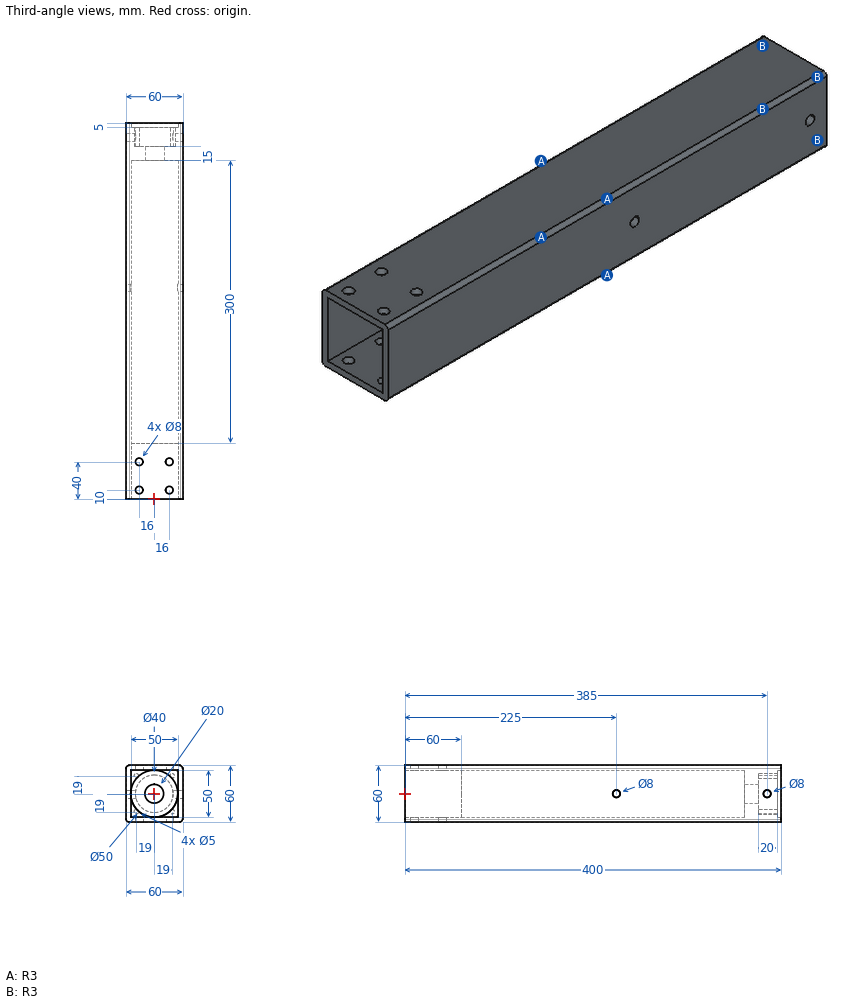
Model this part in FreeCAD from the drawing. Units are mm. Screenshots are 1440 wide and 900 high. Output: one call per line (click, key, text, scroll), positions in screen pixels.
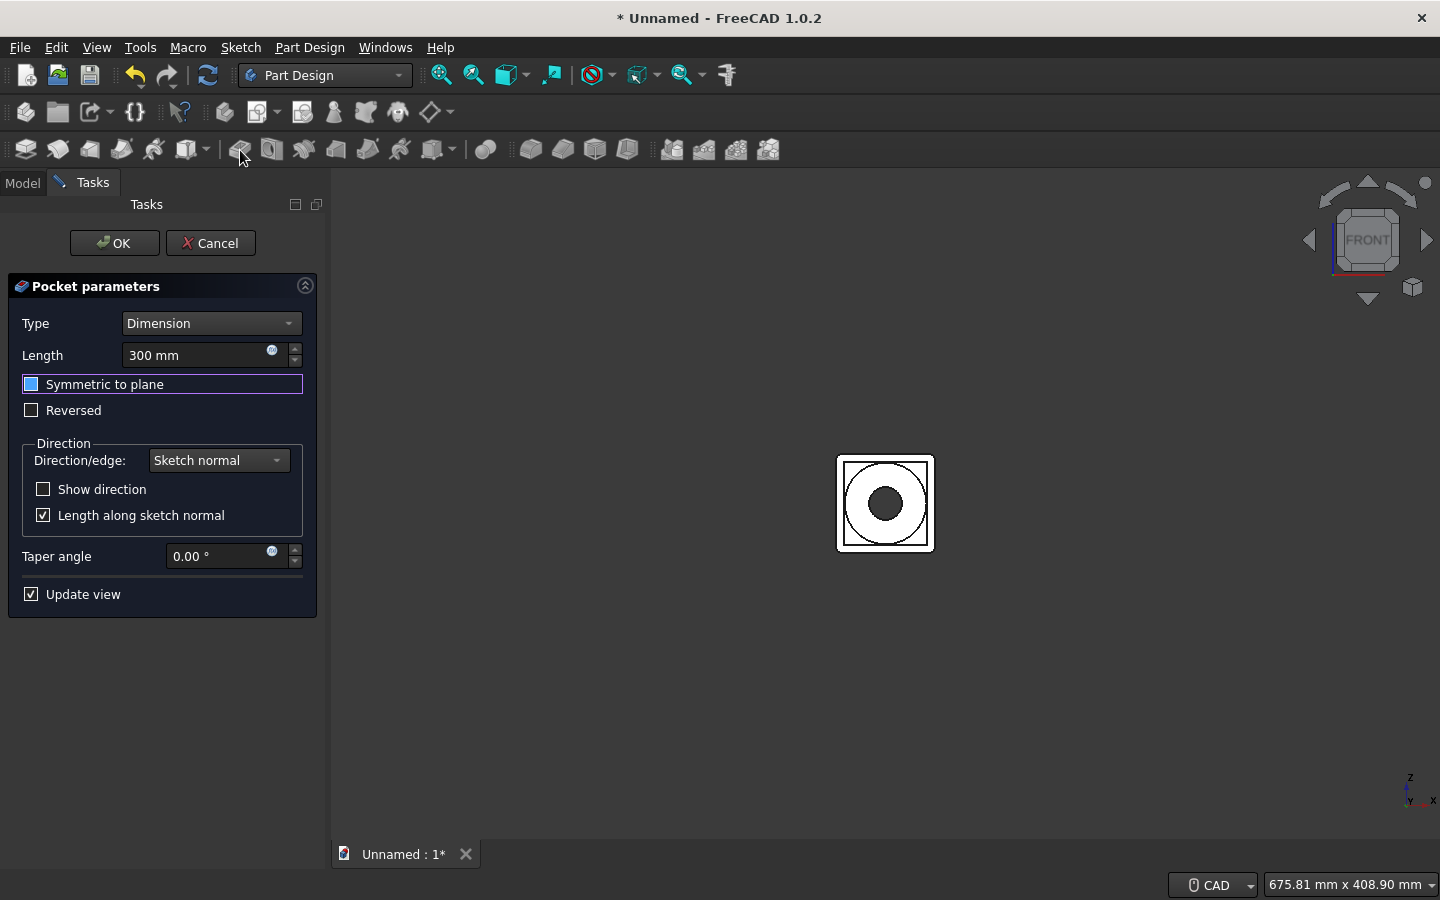
click(115, 243)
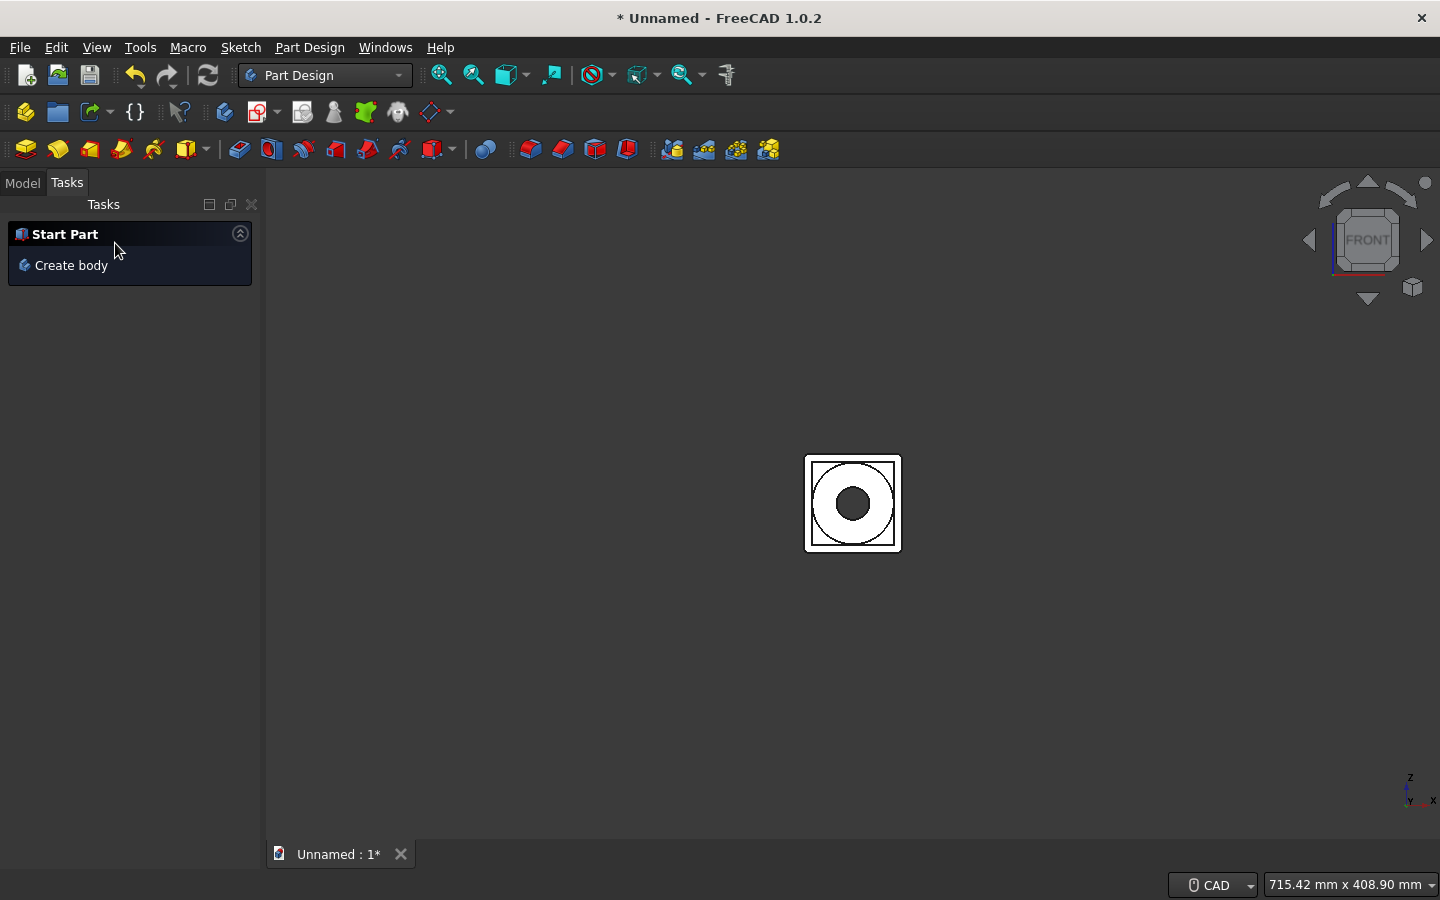
click(442, 76)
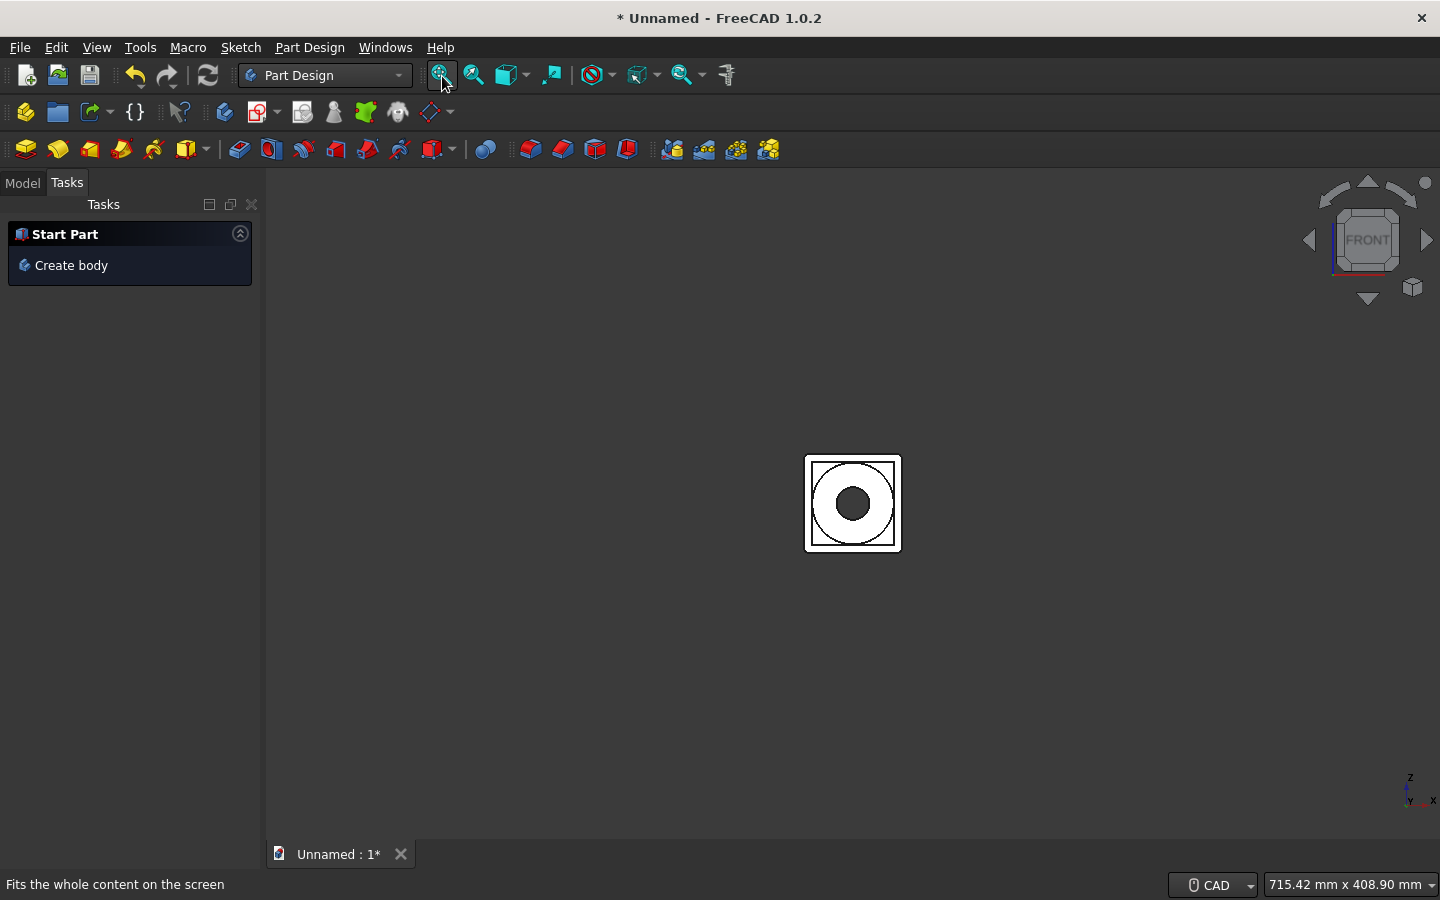
click(258, 112)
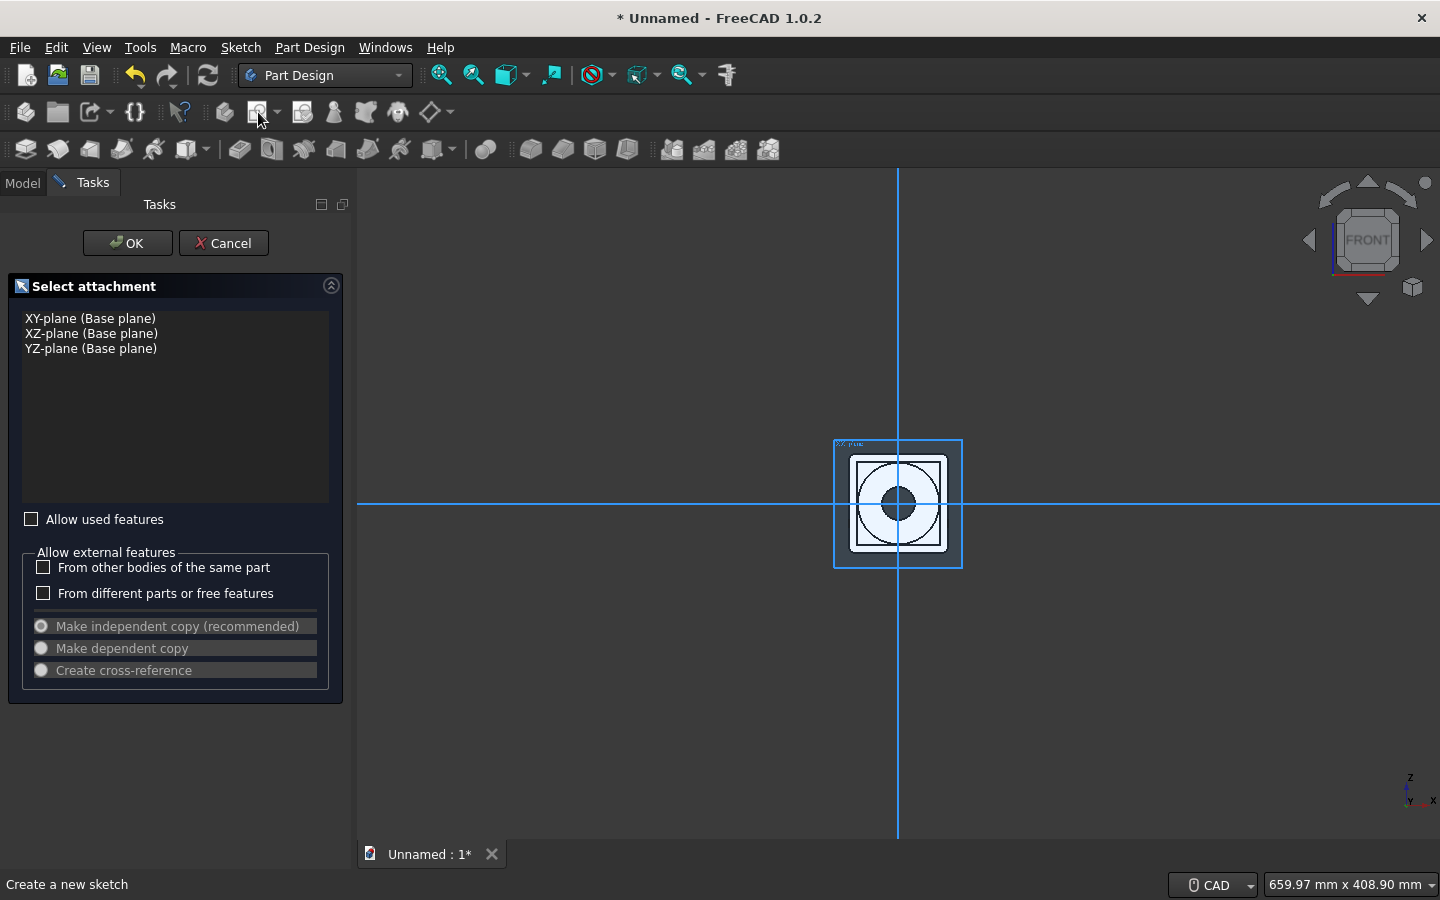
click(82, 348)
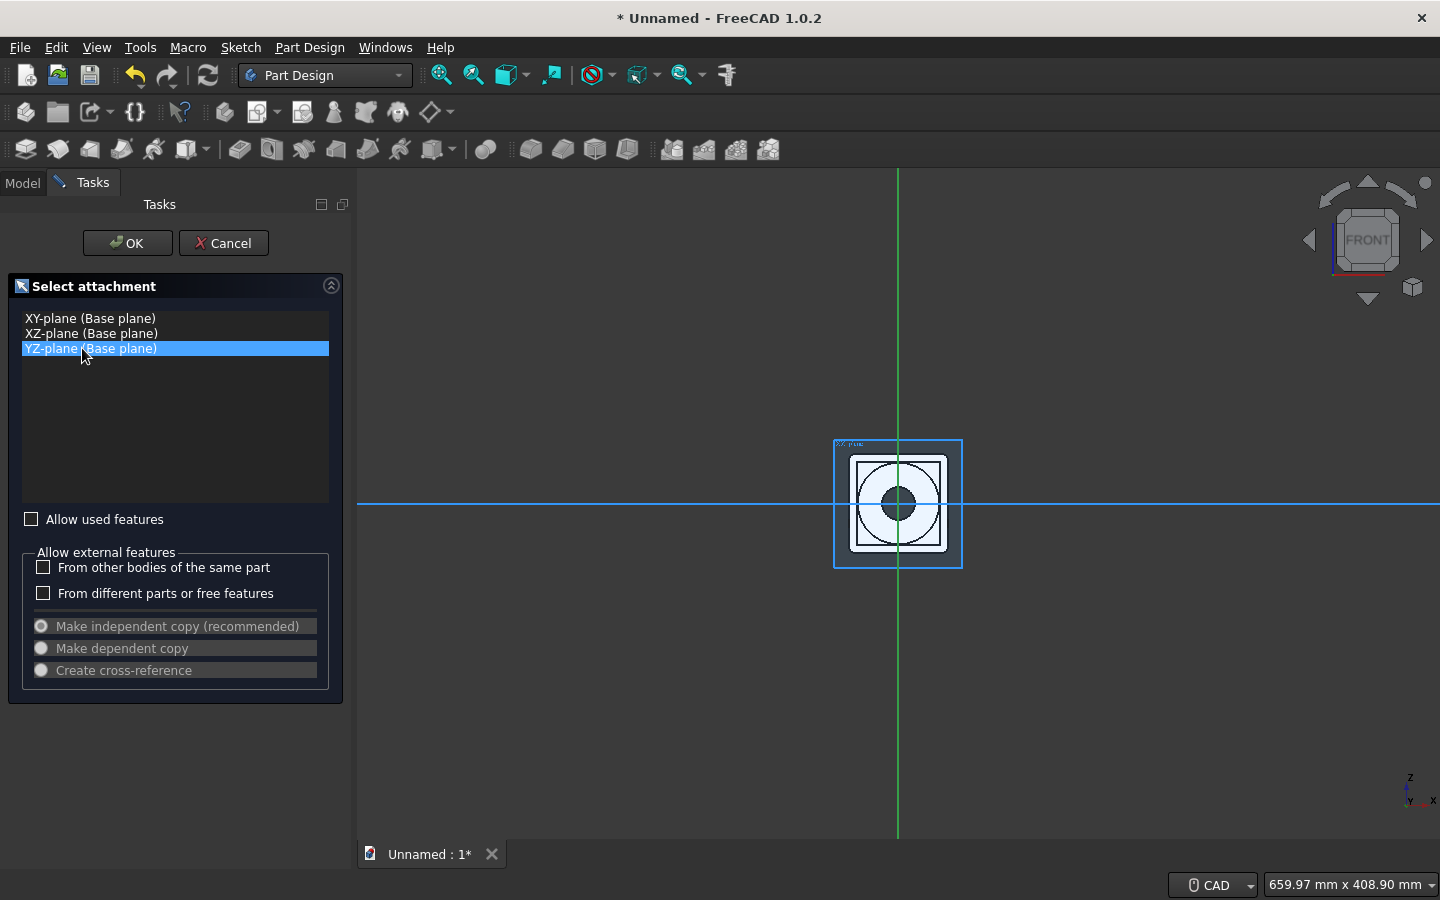
click(128, 243)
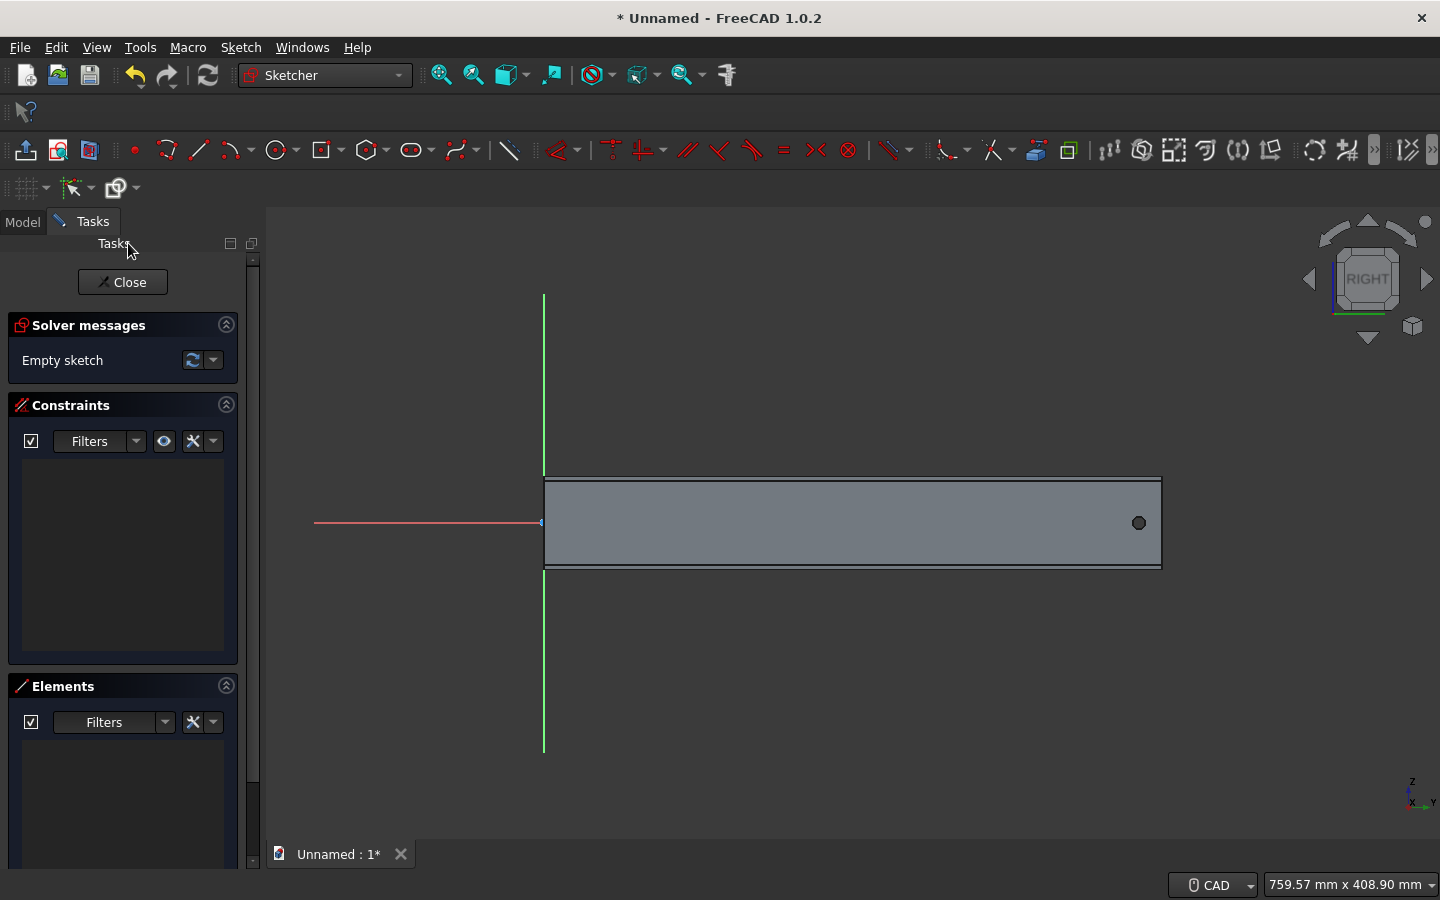
click(90, 150)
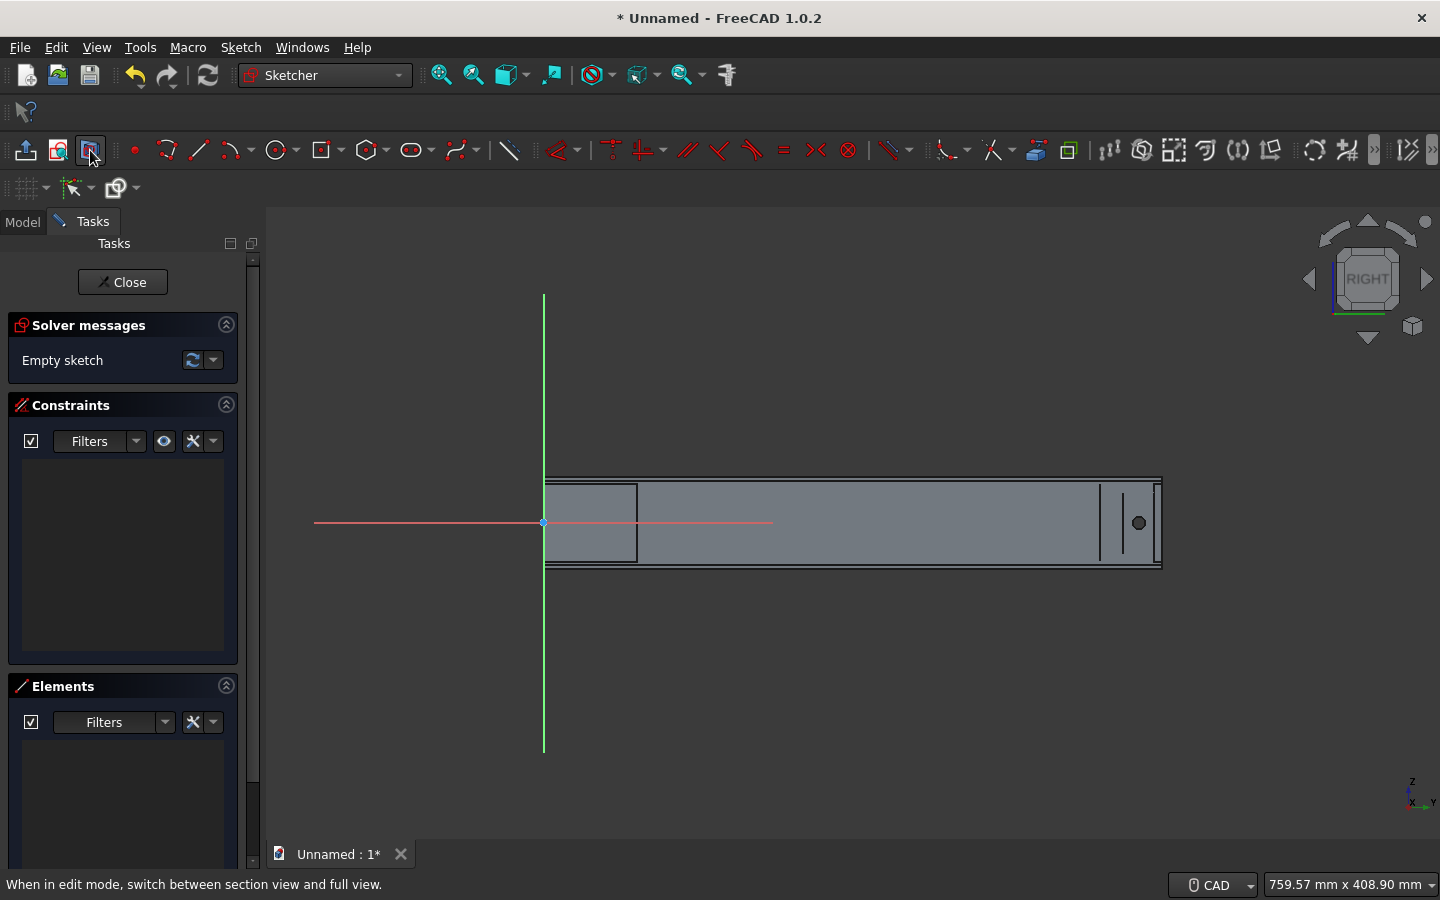
scroll(897, 523, up, 15)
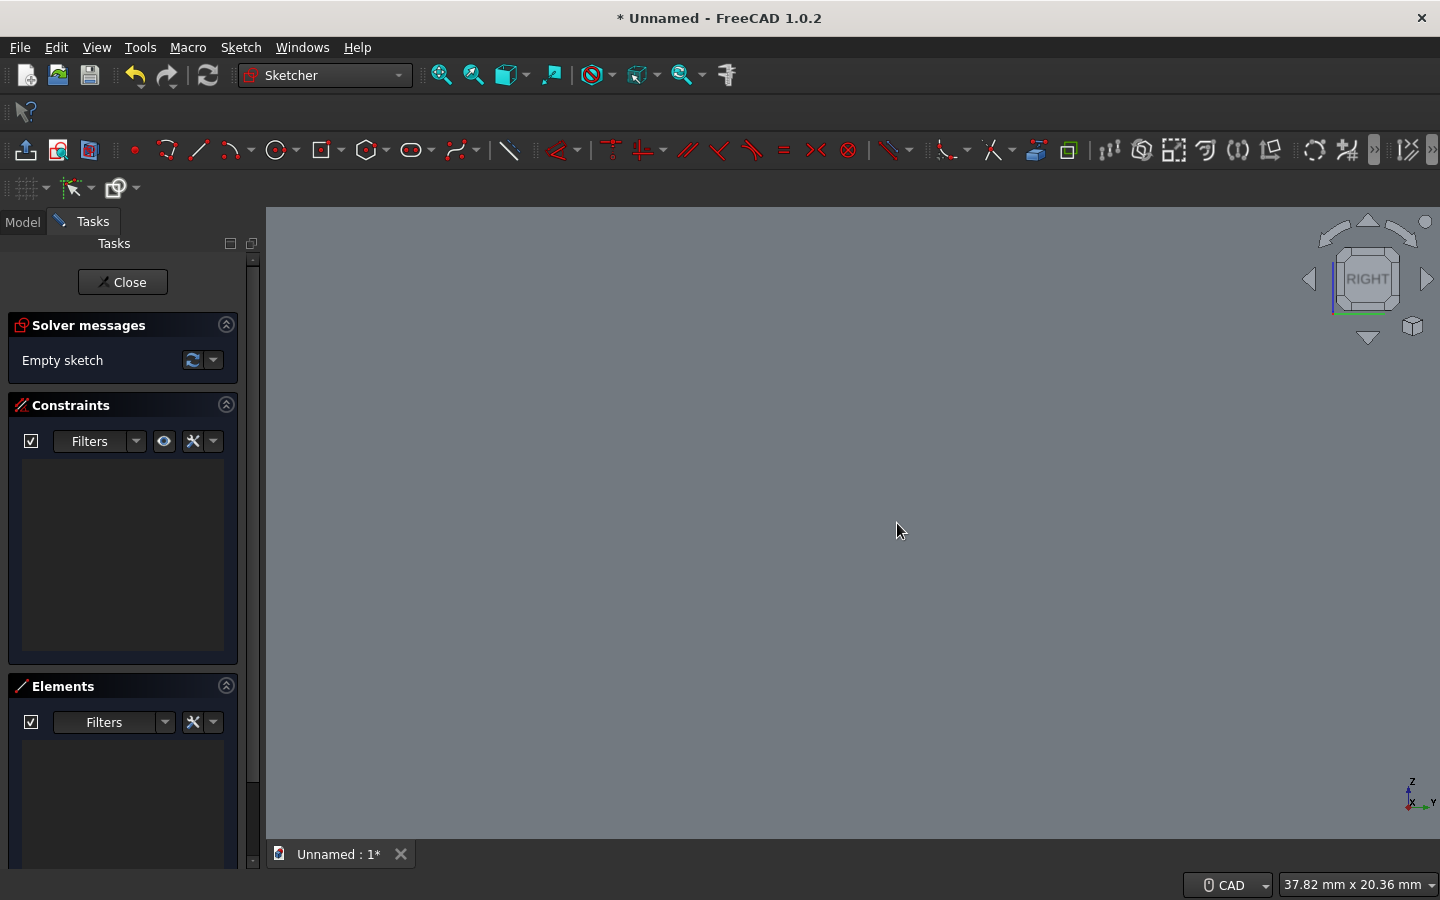
scroll(768, 494, up, 2)